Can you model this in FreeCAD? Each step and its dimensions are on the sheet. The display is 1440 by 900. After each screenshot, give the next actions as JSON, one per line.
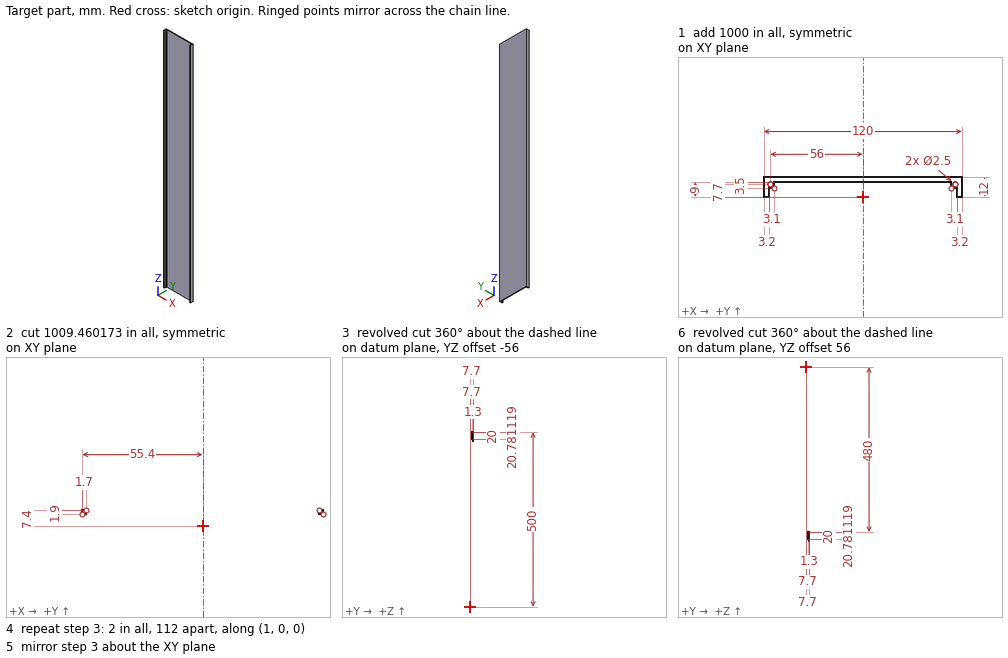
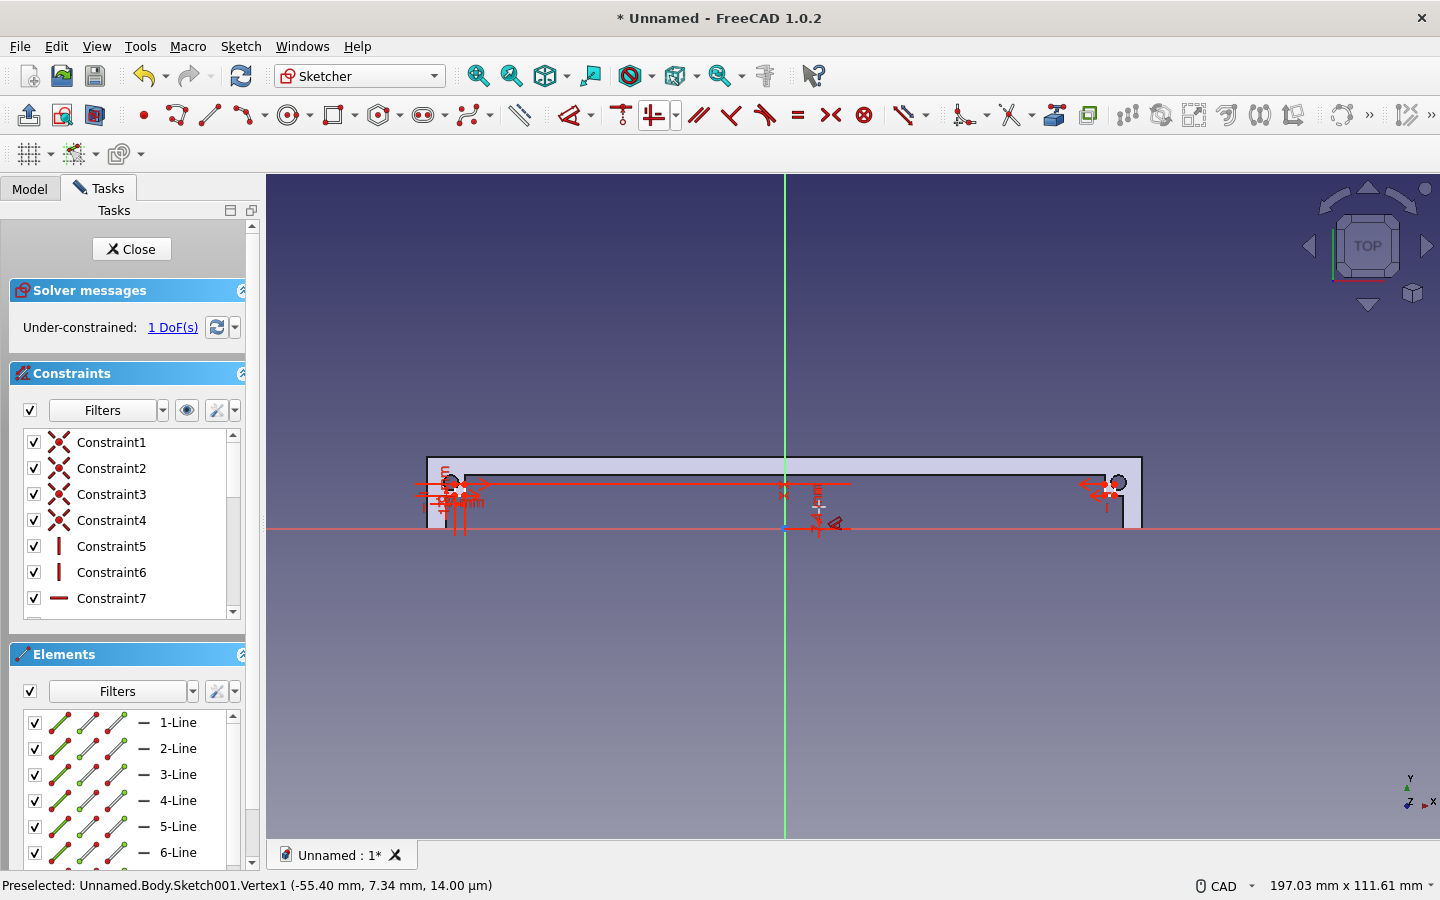
{"action": "left_click", "coordinate": [455, 484]}
{"action": "left_click", "coordinate": [620, 563]}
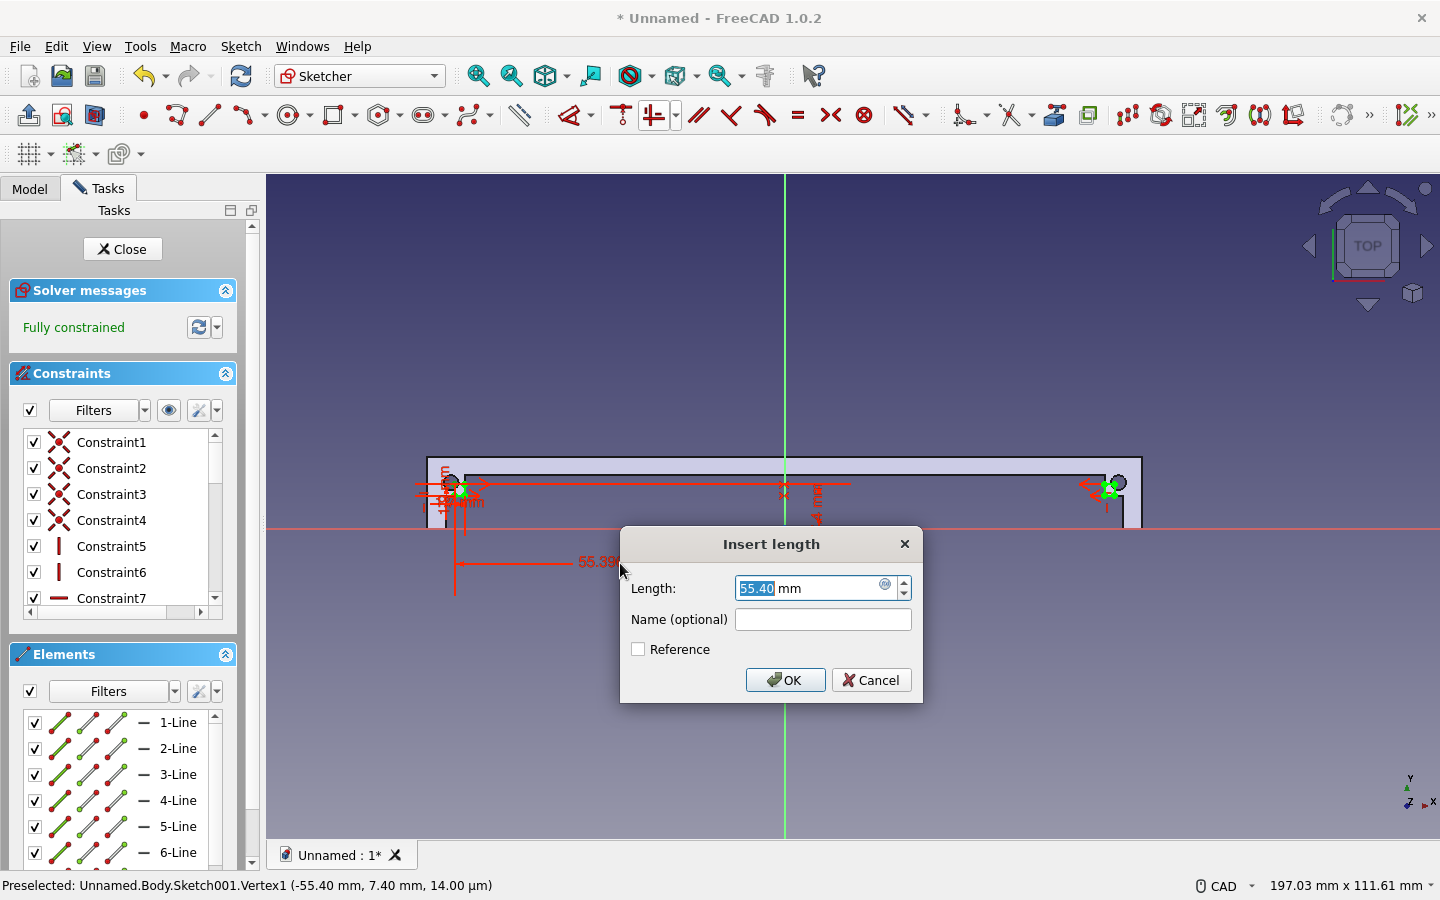
{"action": "type", "text": "55.4"}
{"action": "key", "text": "Return"}
{"action": "key", "text": "Escape"}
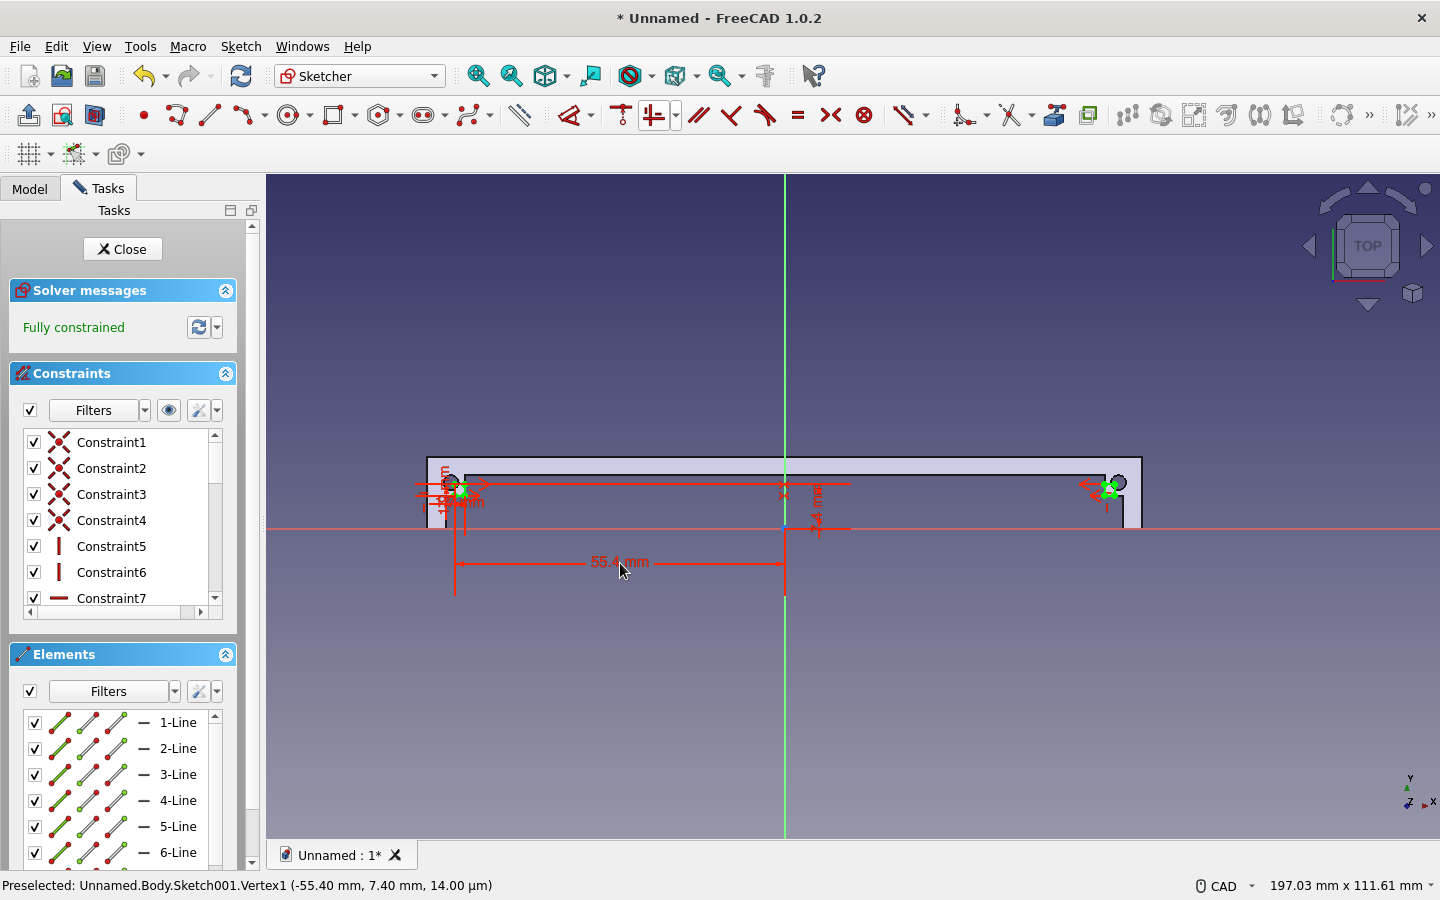
{"action": "left_click", "coordinate": [123, 249]}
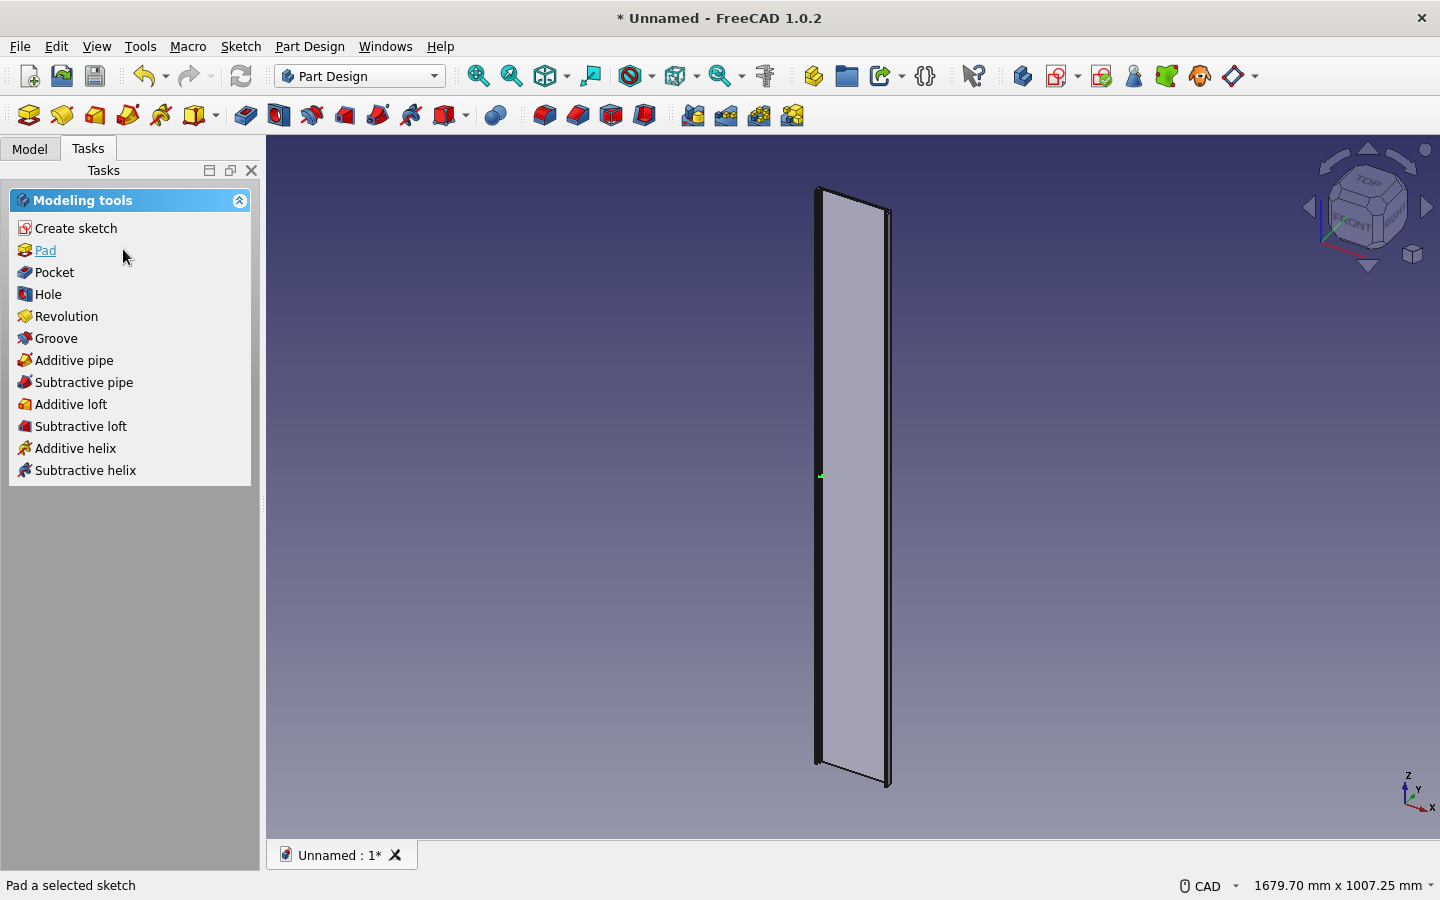
{"action": "left_click", "coordinate": [246, 116]}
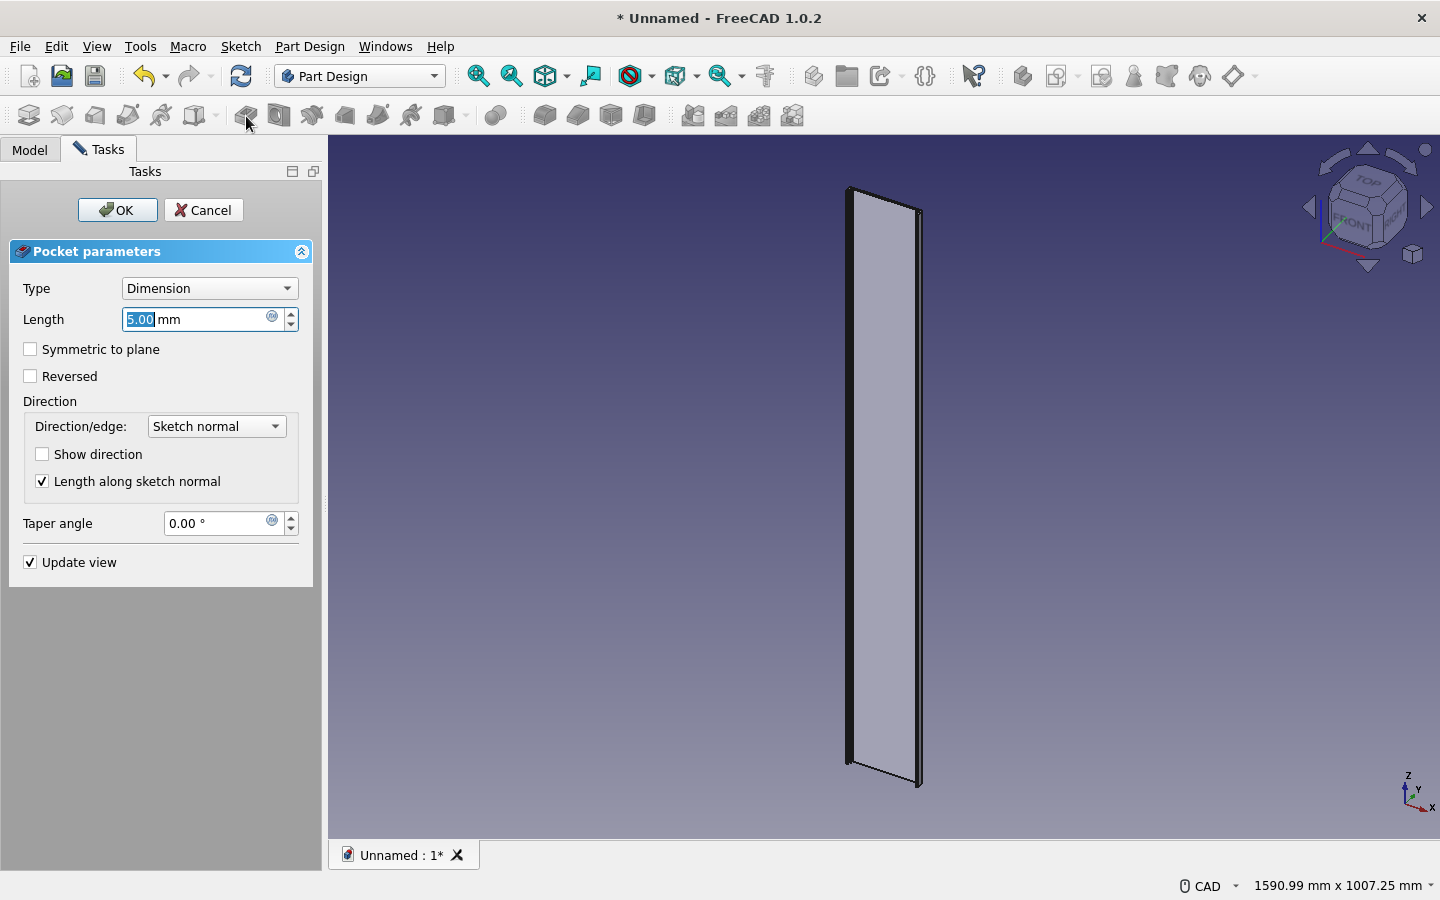
{"action": "type", "text": "1009.460173"}
{"action": "key", "text": "Tab"}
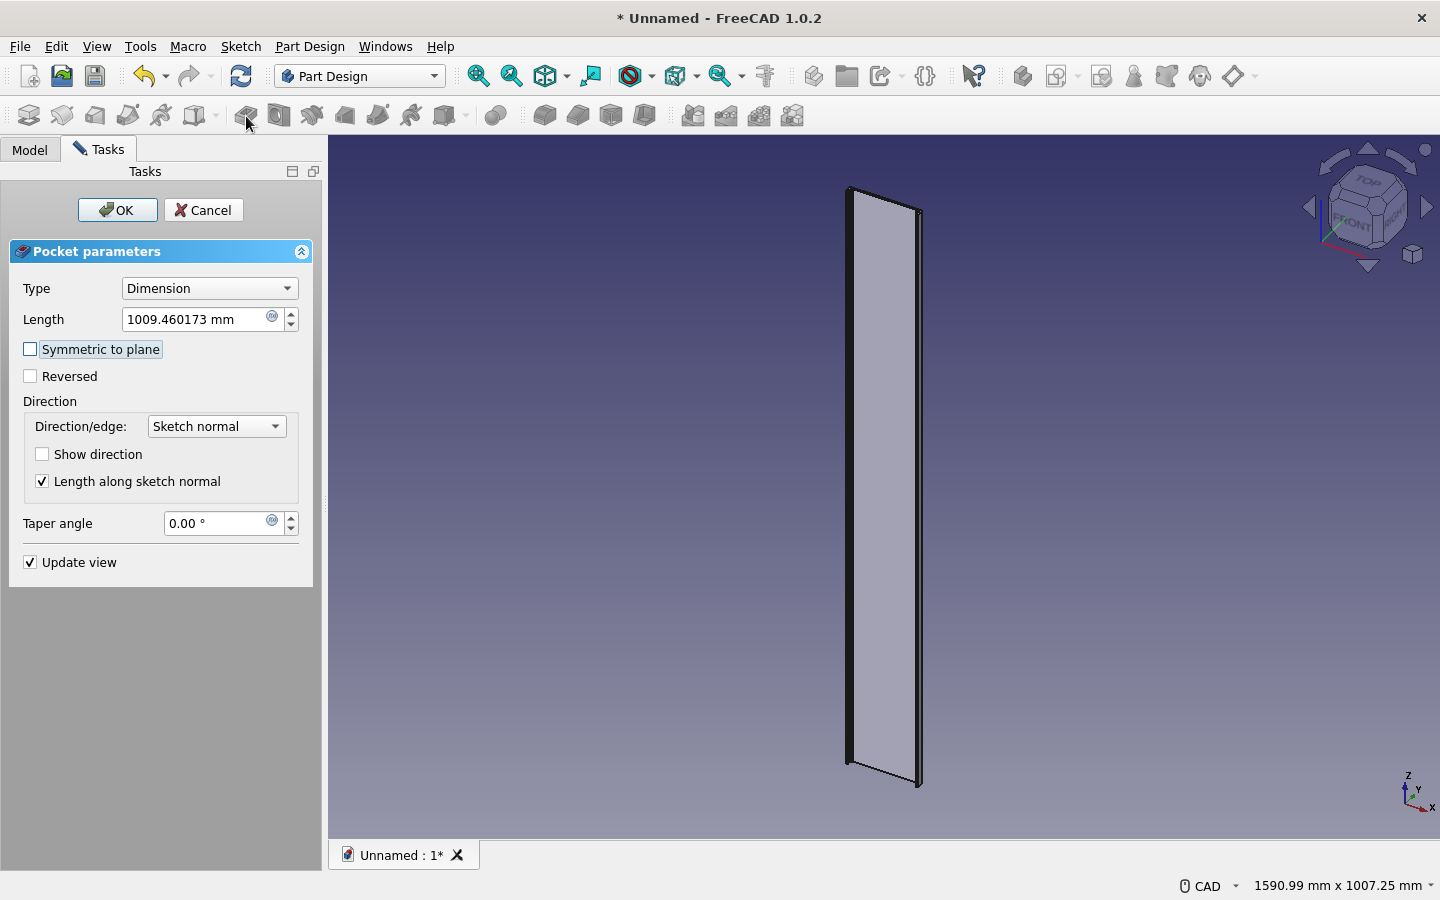
{"action": "left_click", "coordinate": [31, 349]}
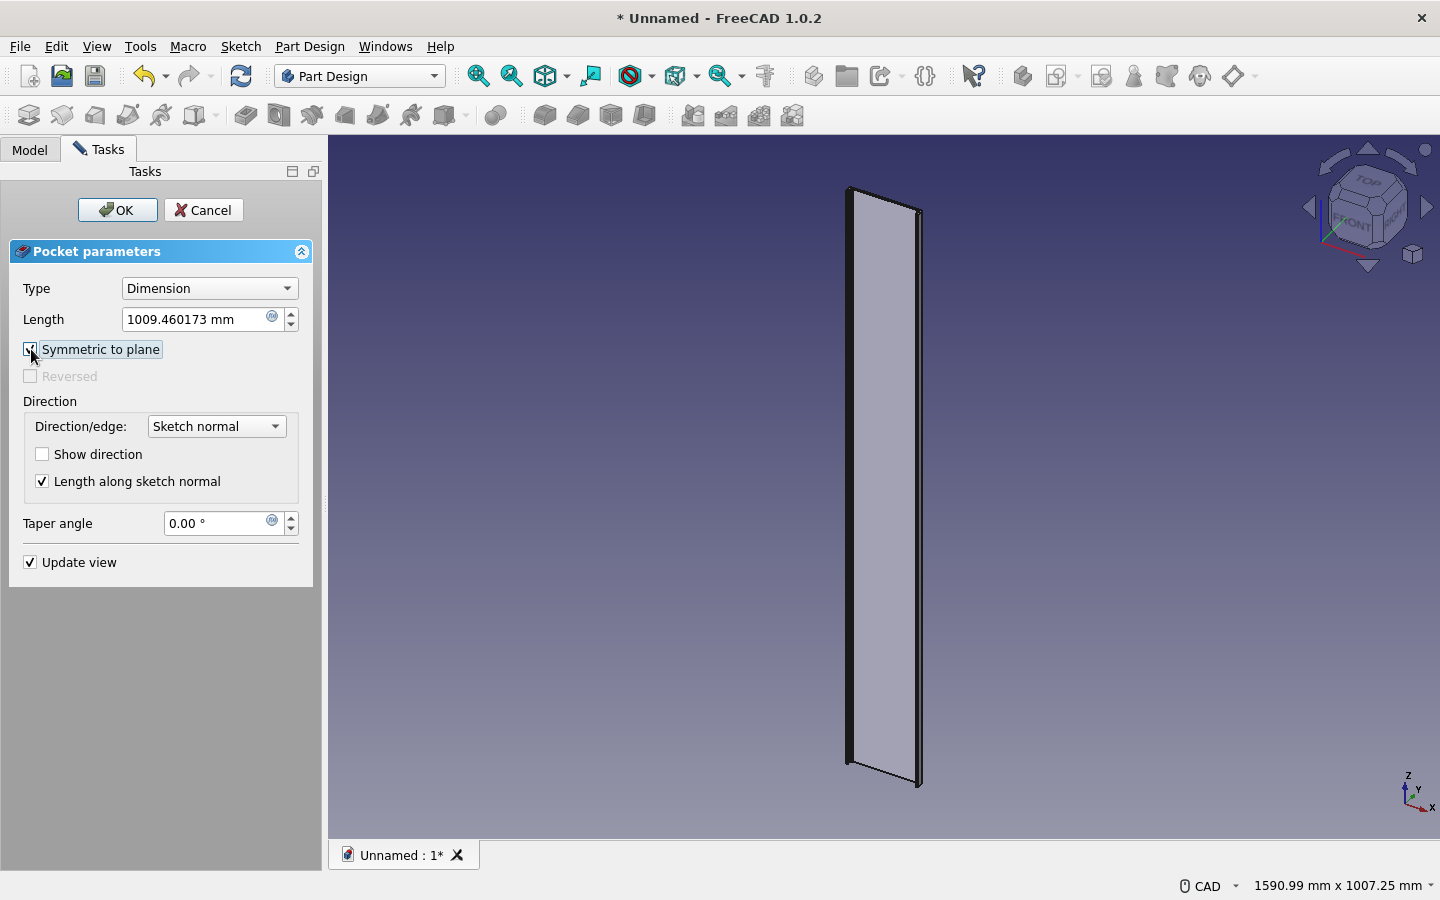
{"action": "left_click", "coordinate": [118, 210]}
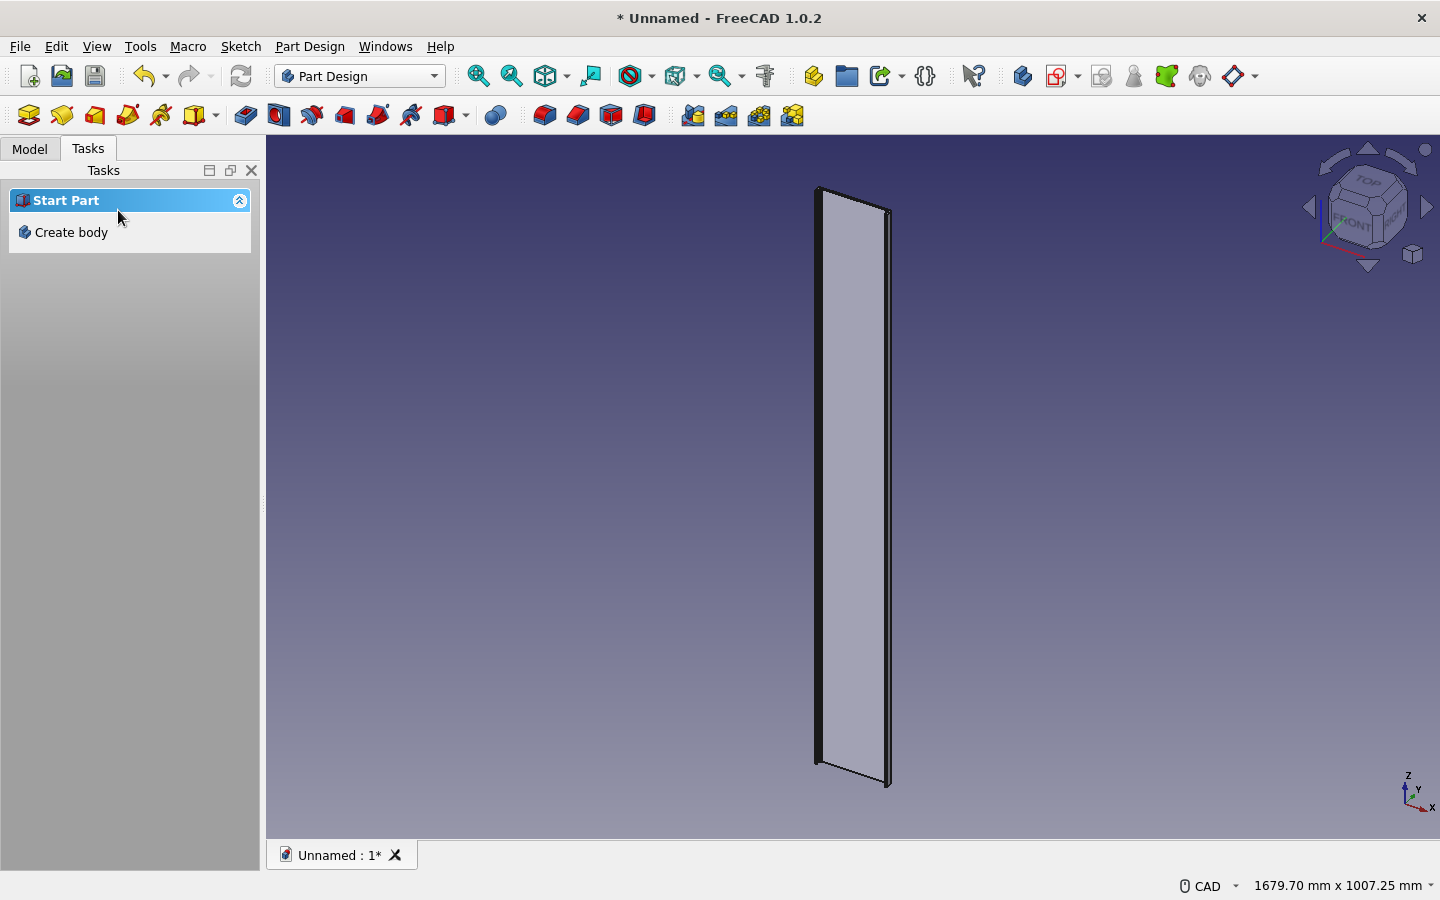
{"action": "left_click", "coordinate": [30, 148]}